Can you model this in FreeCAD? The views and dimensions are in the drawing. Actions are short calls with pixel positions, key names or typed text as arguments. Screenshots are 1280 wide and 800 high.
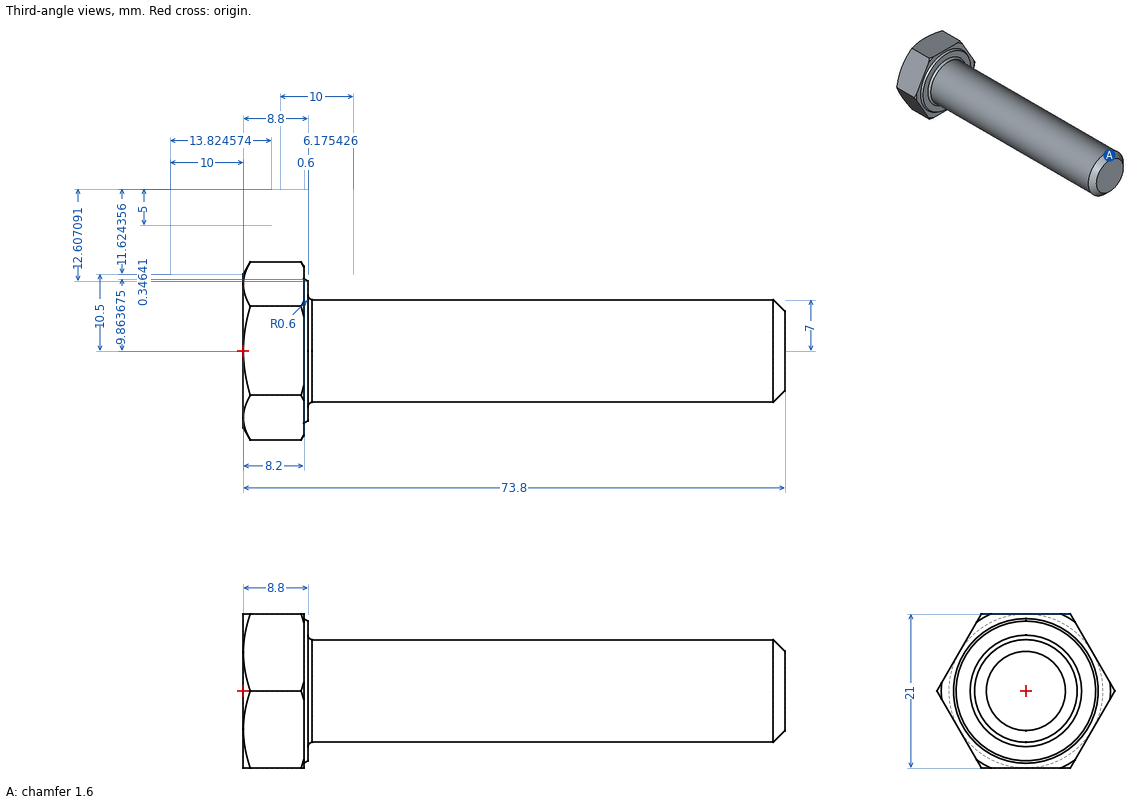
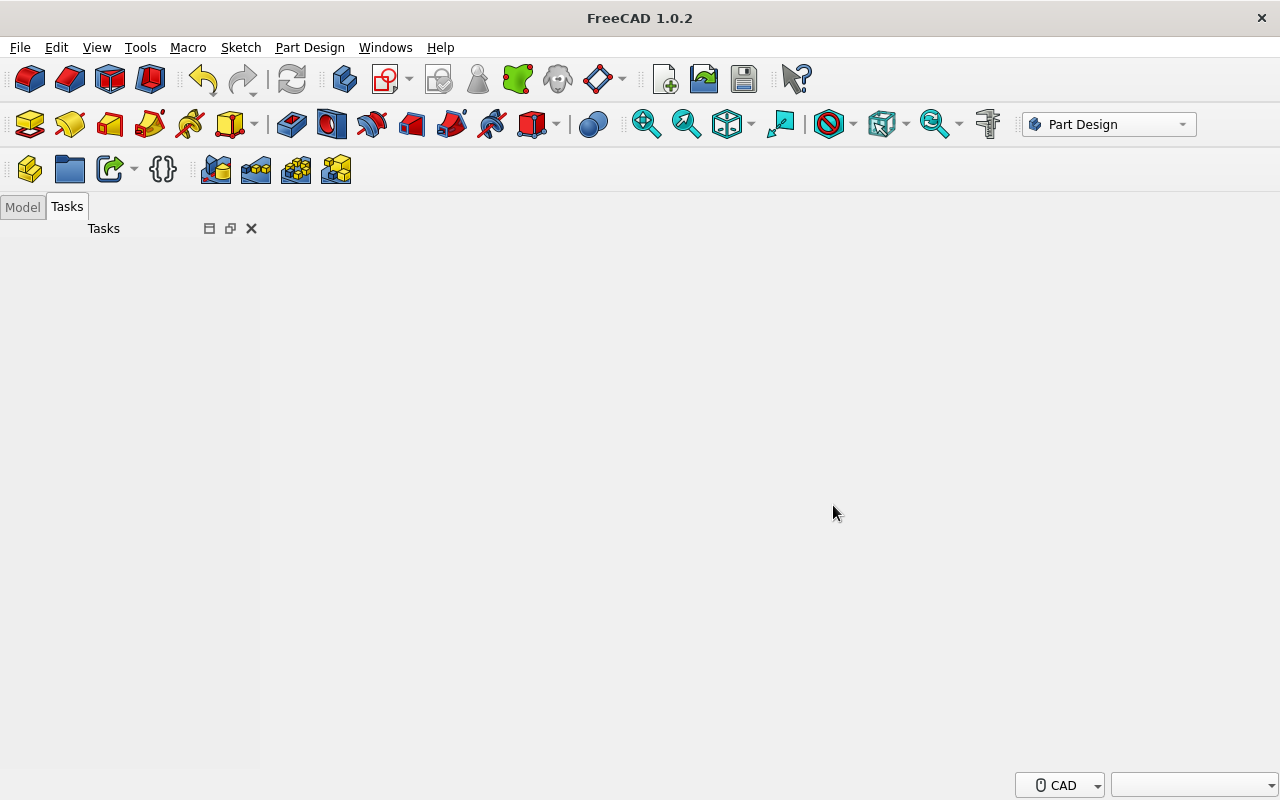
click(664, 80)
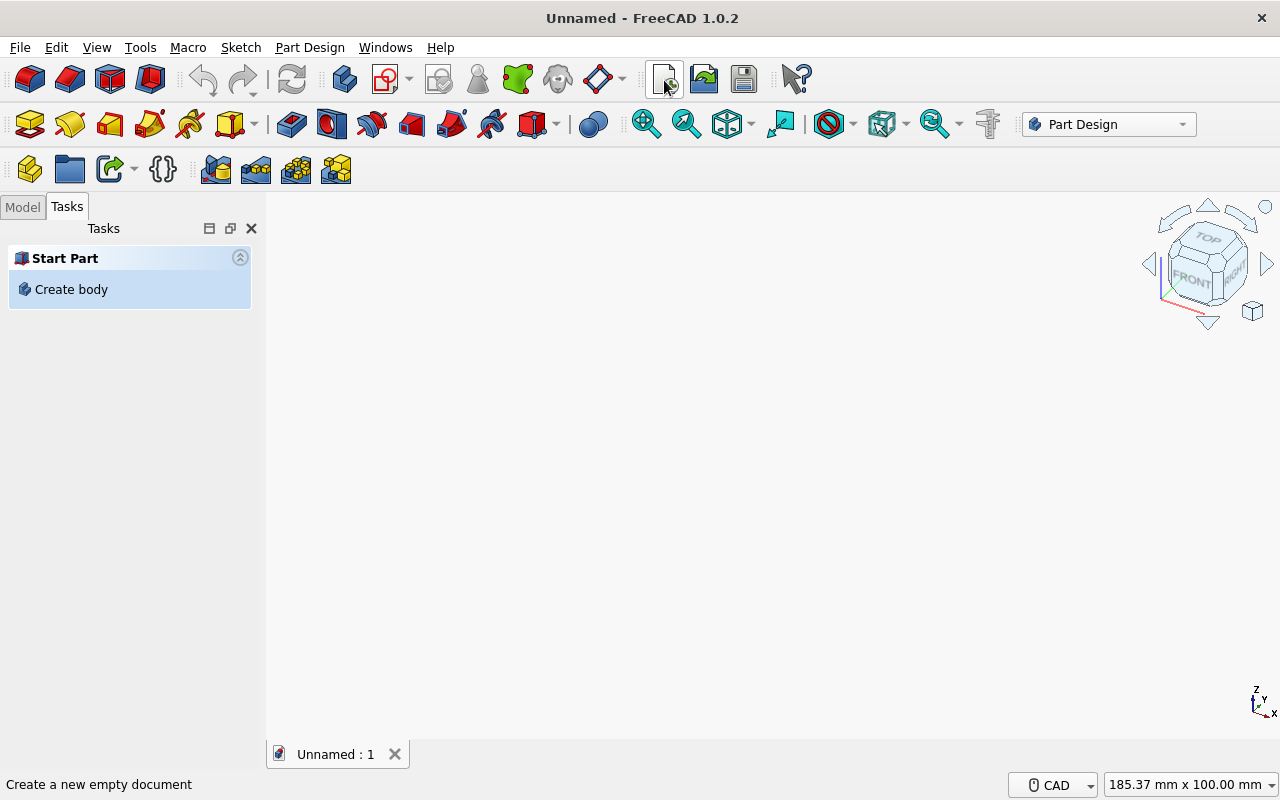
click(386, 80)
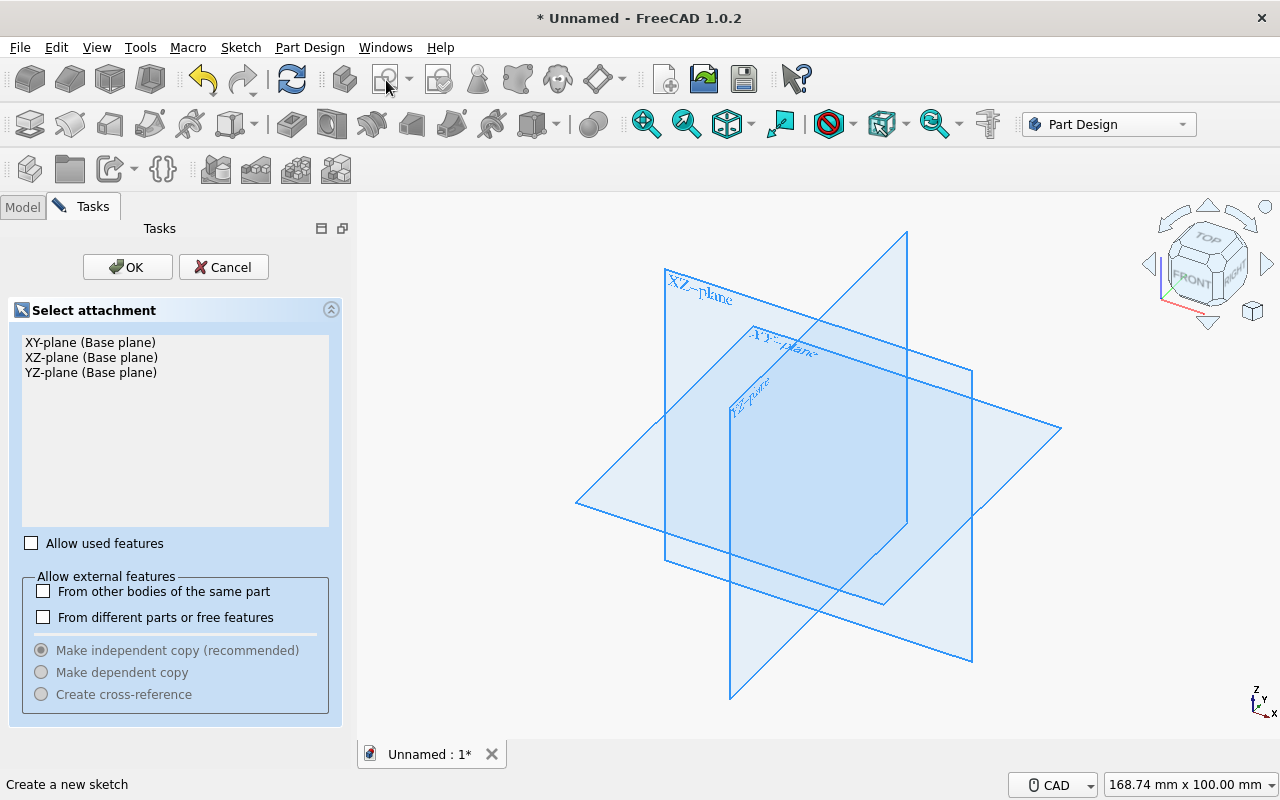
click(82, 372)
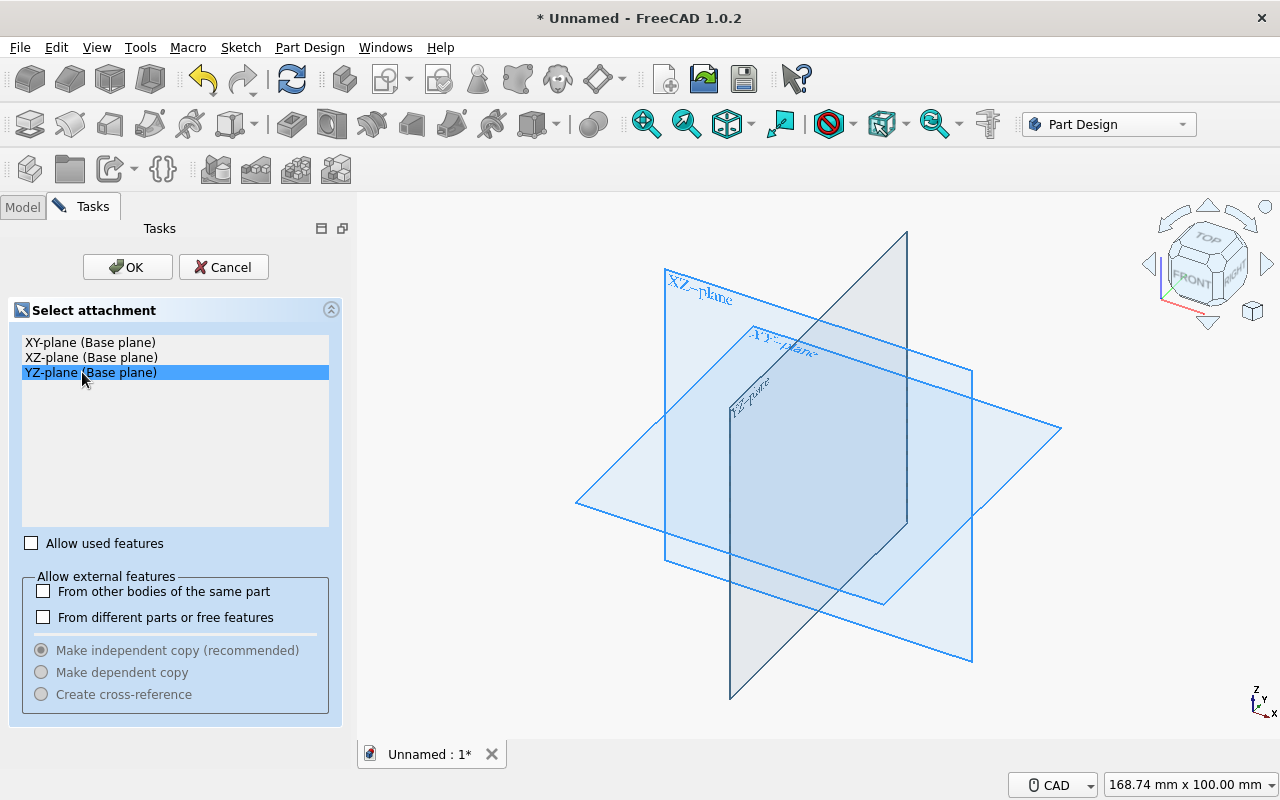
click(128, 267)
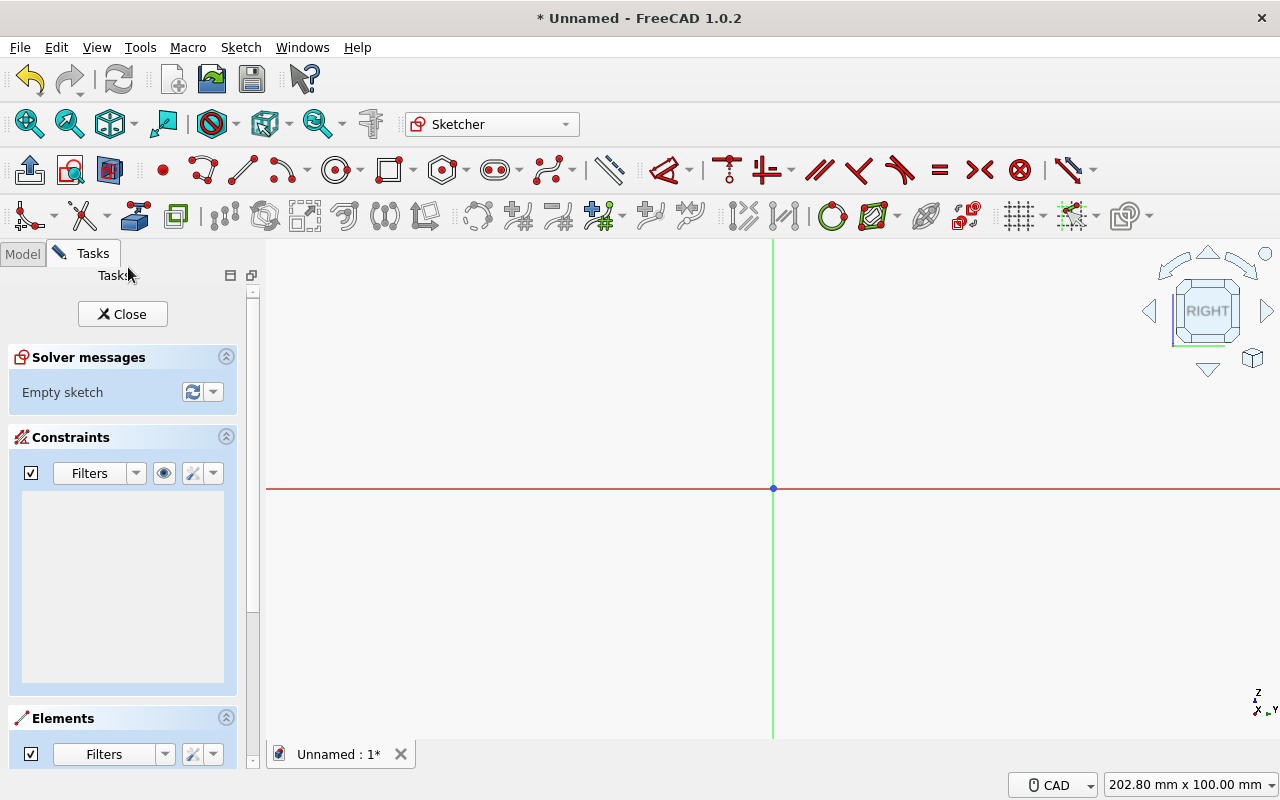
scroll(813, 489, up, 5)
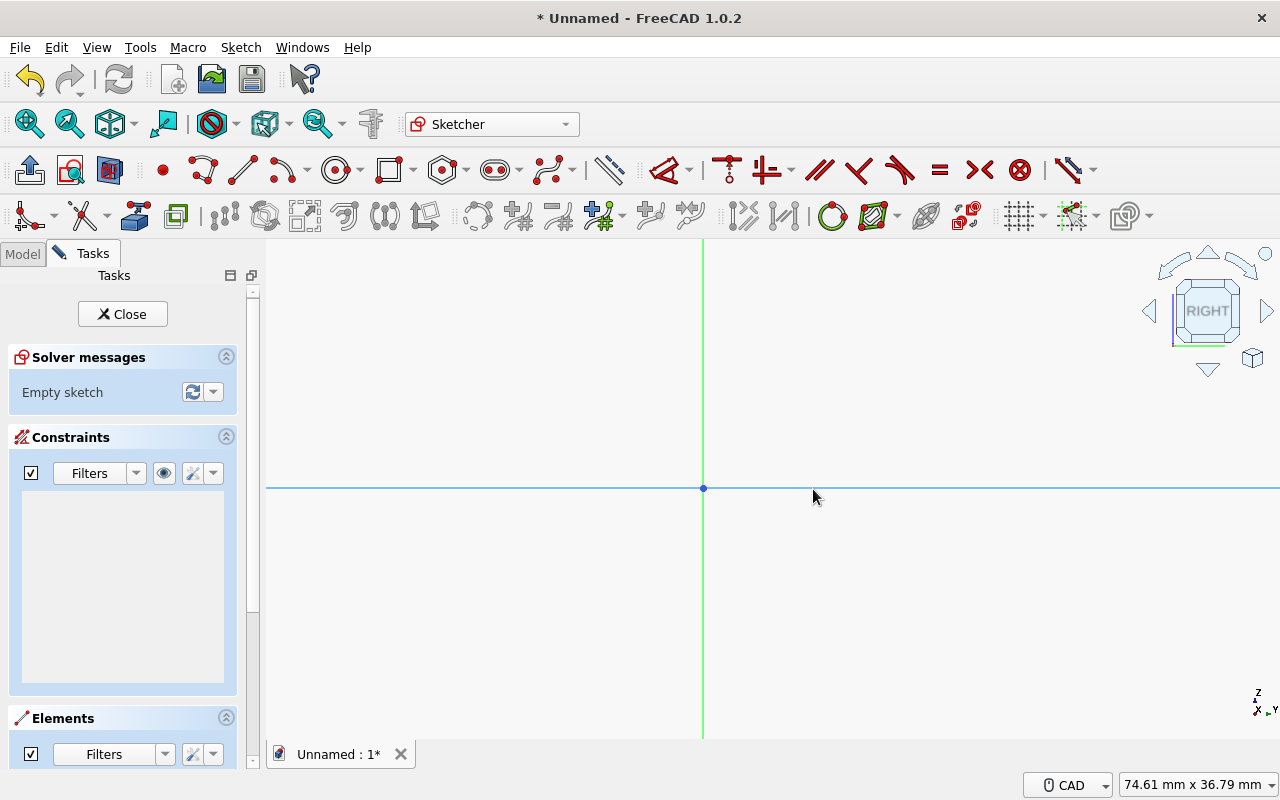
click(442, 170)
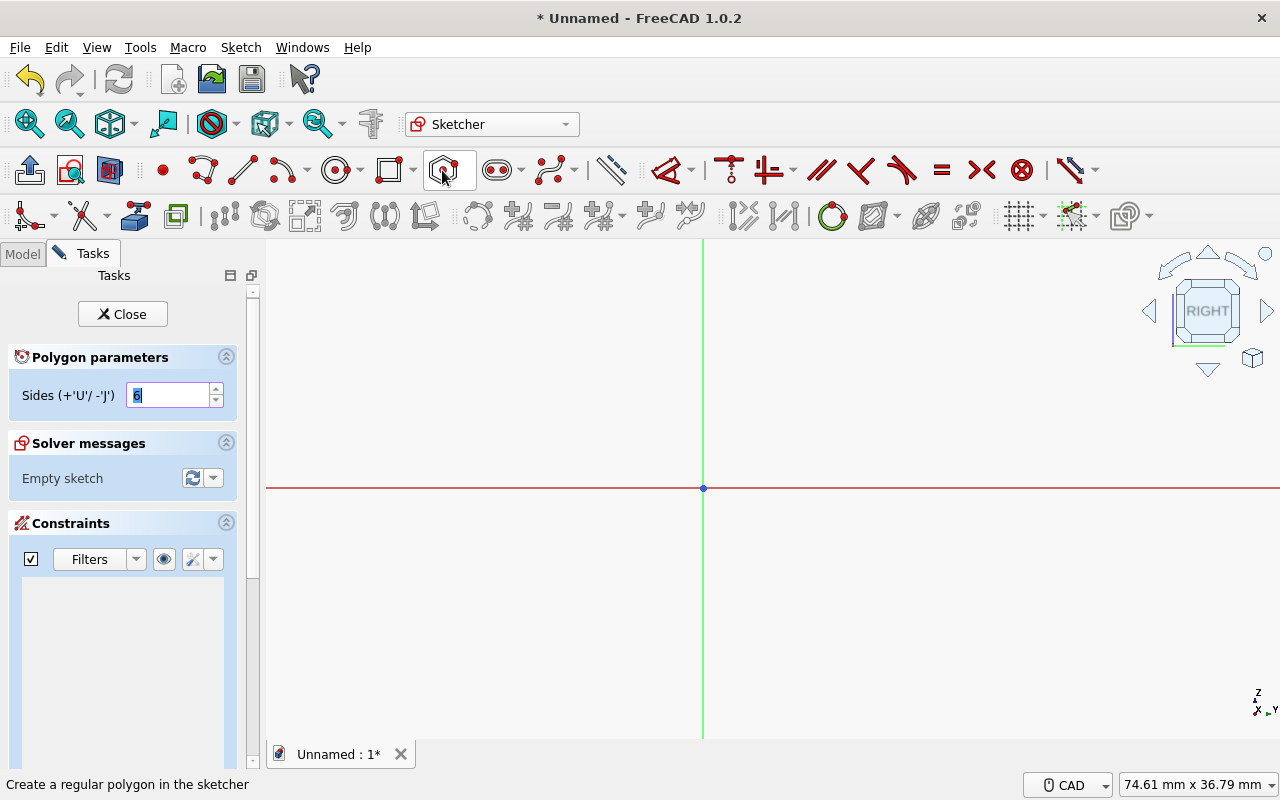
click(703, 488)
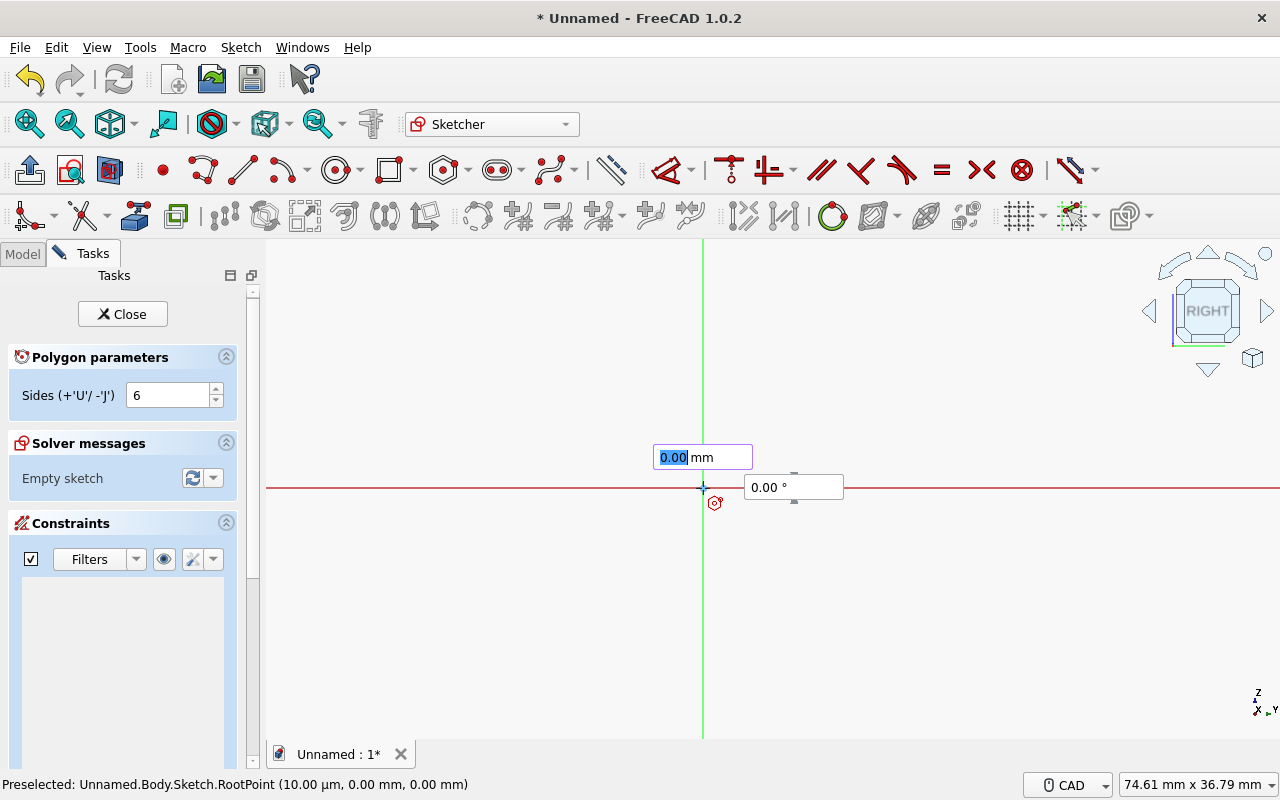
click(868, 488)
key(Escape)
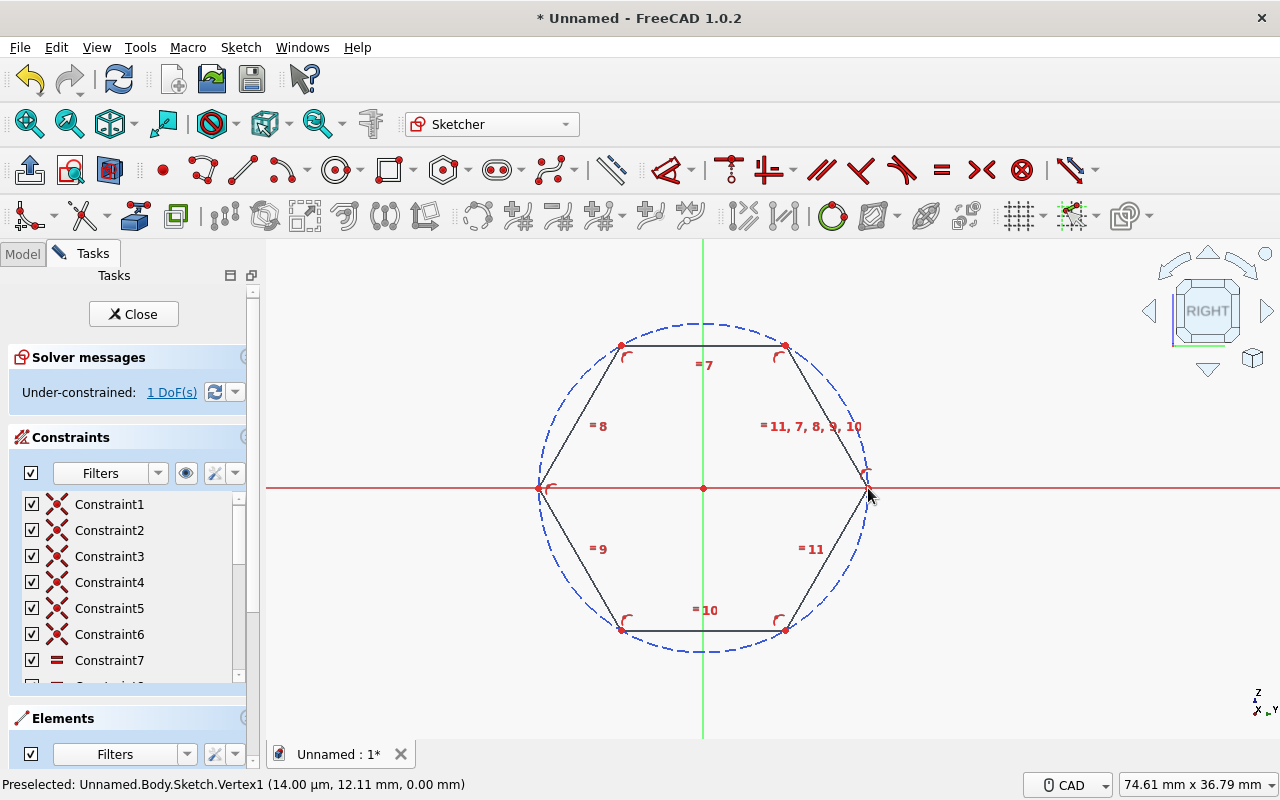
click(666, 170)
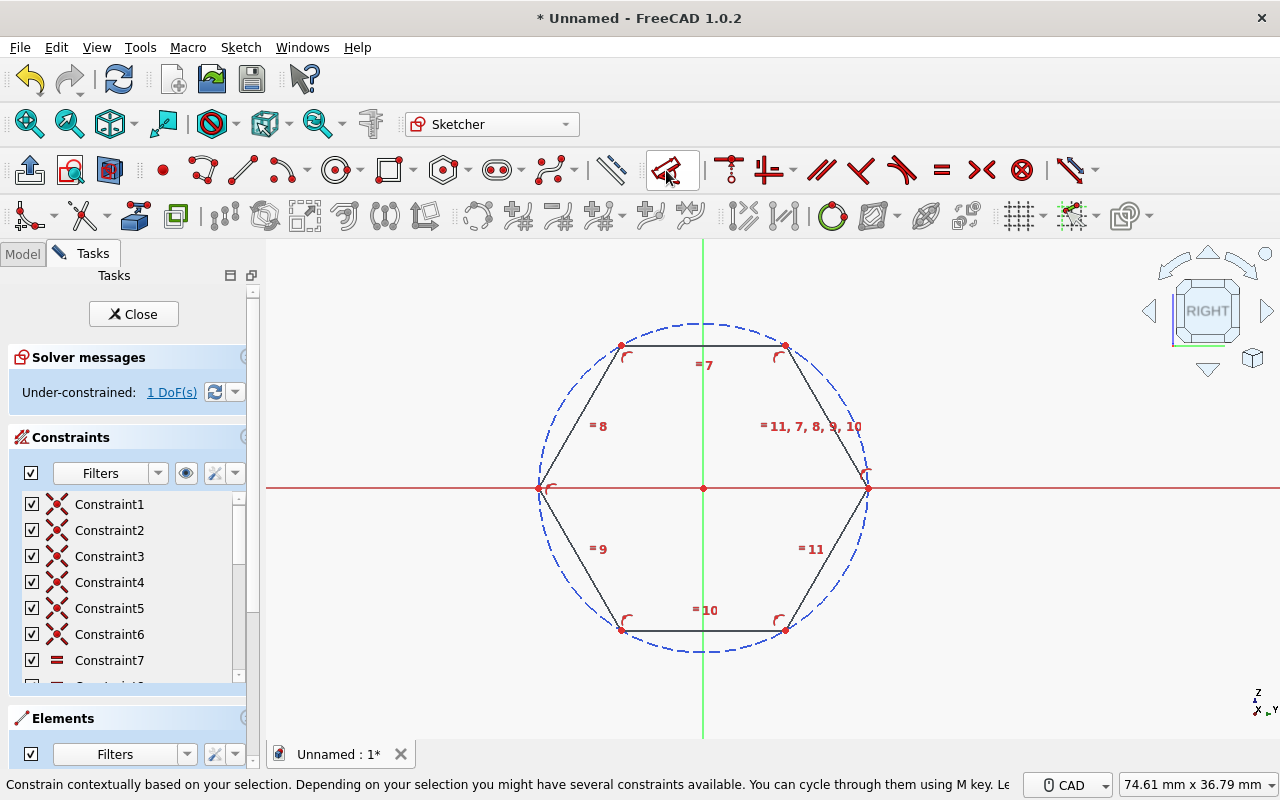
click(621, 631)